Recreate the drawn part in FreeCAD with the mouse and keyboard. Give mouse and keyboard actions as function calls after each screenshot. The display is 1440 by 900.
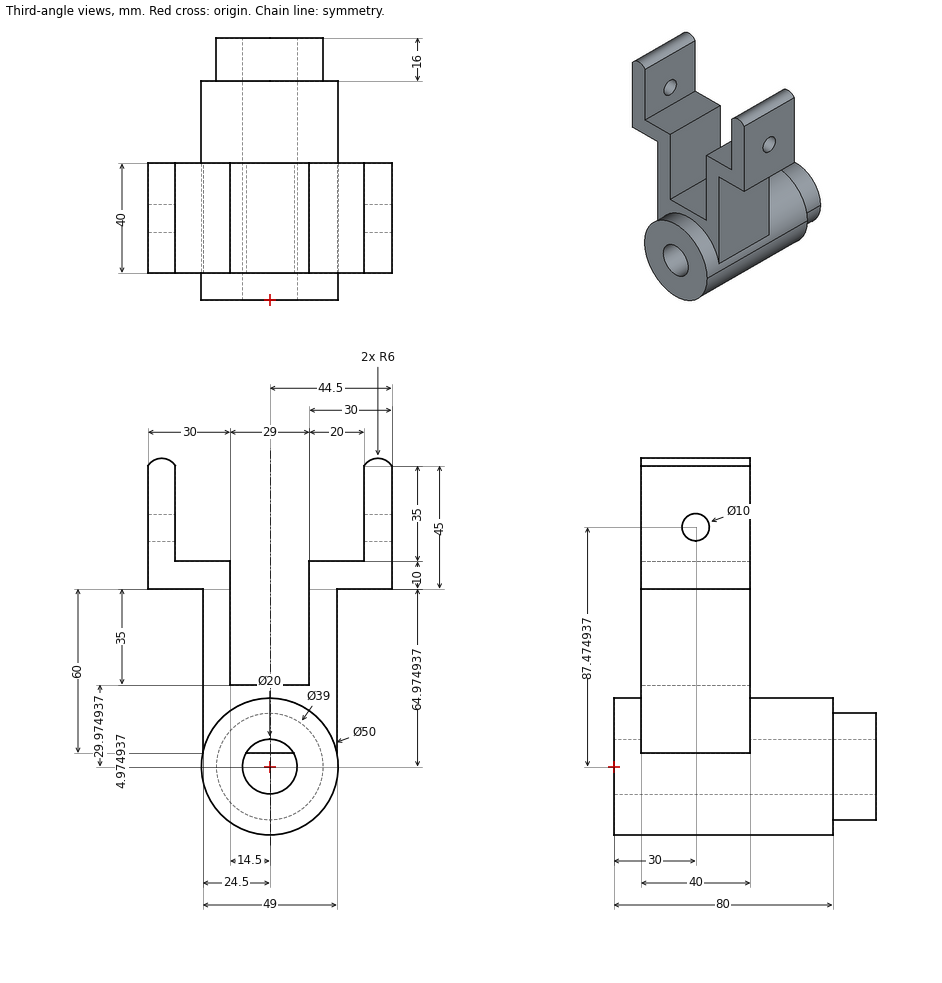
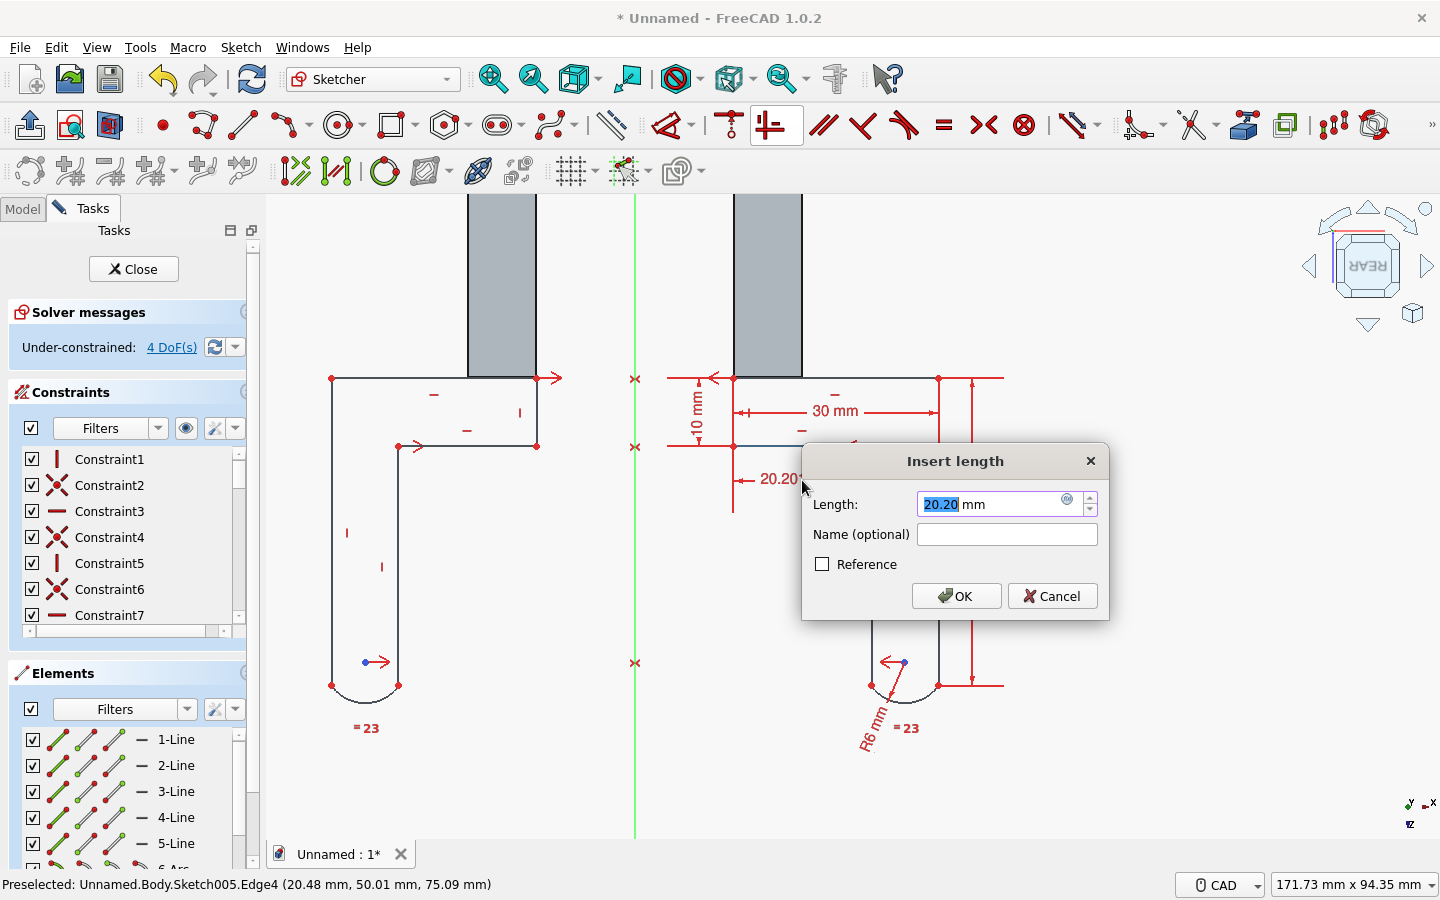
text(20)
key(Return)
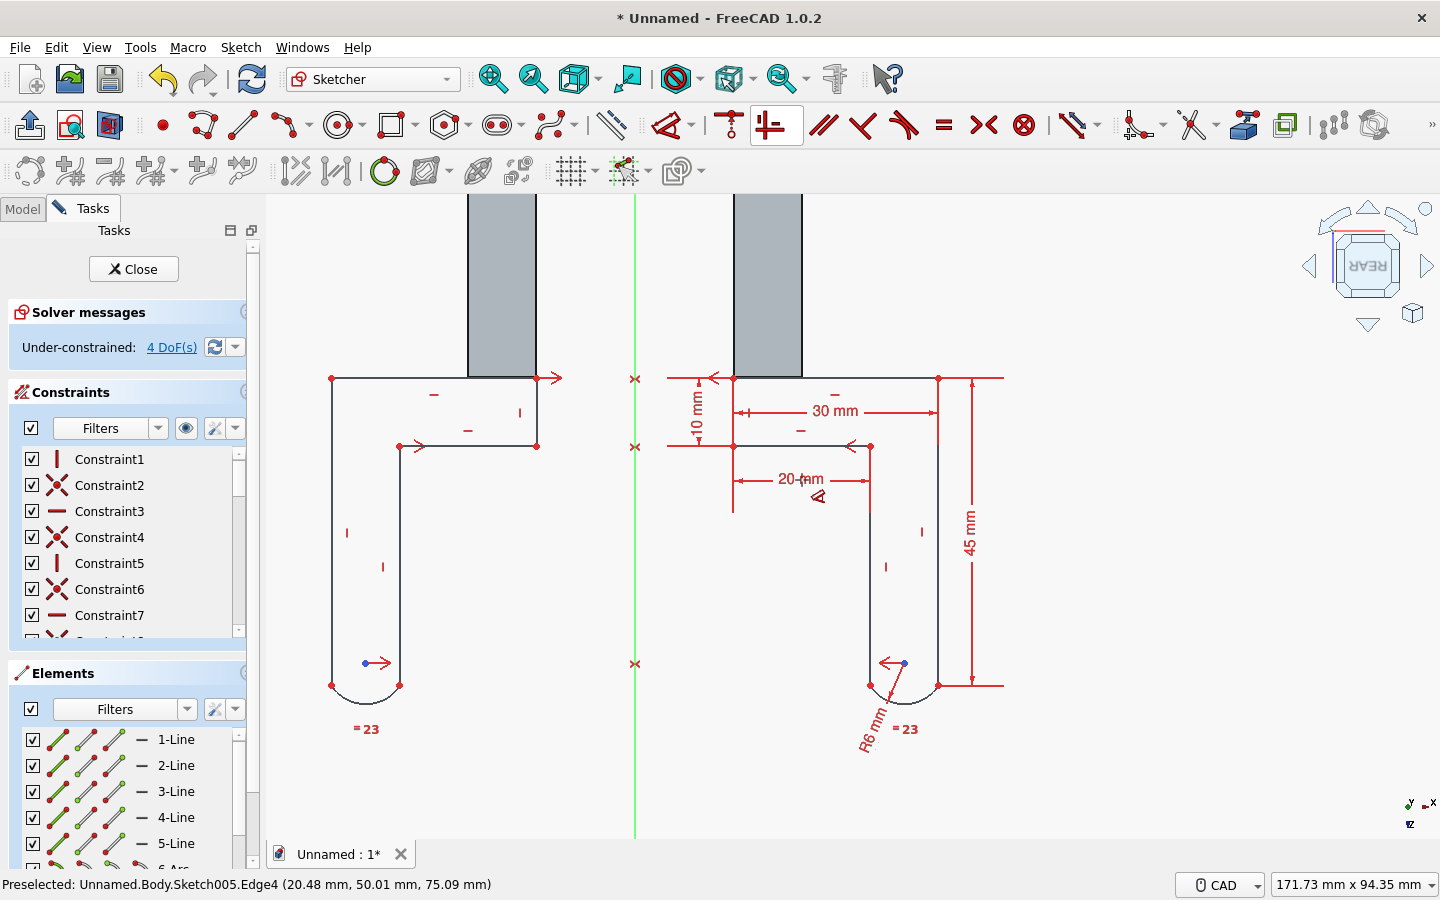
click(870, 518)
click(904, 566)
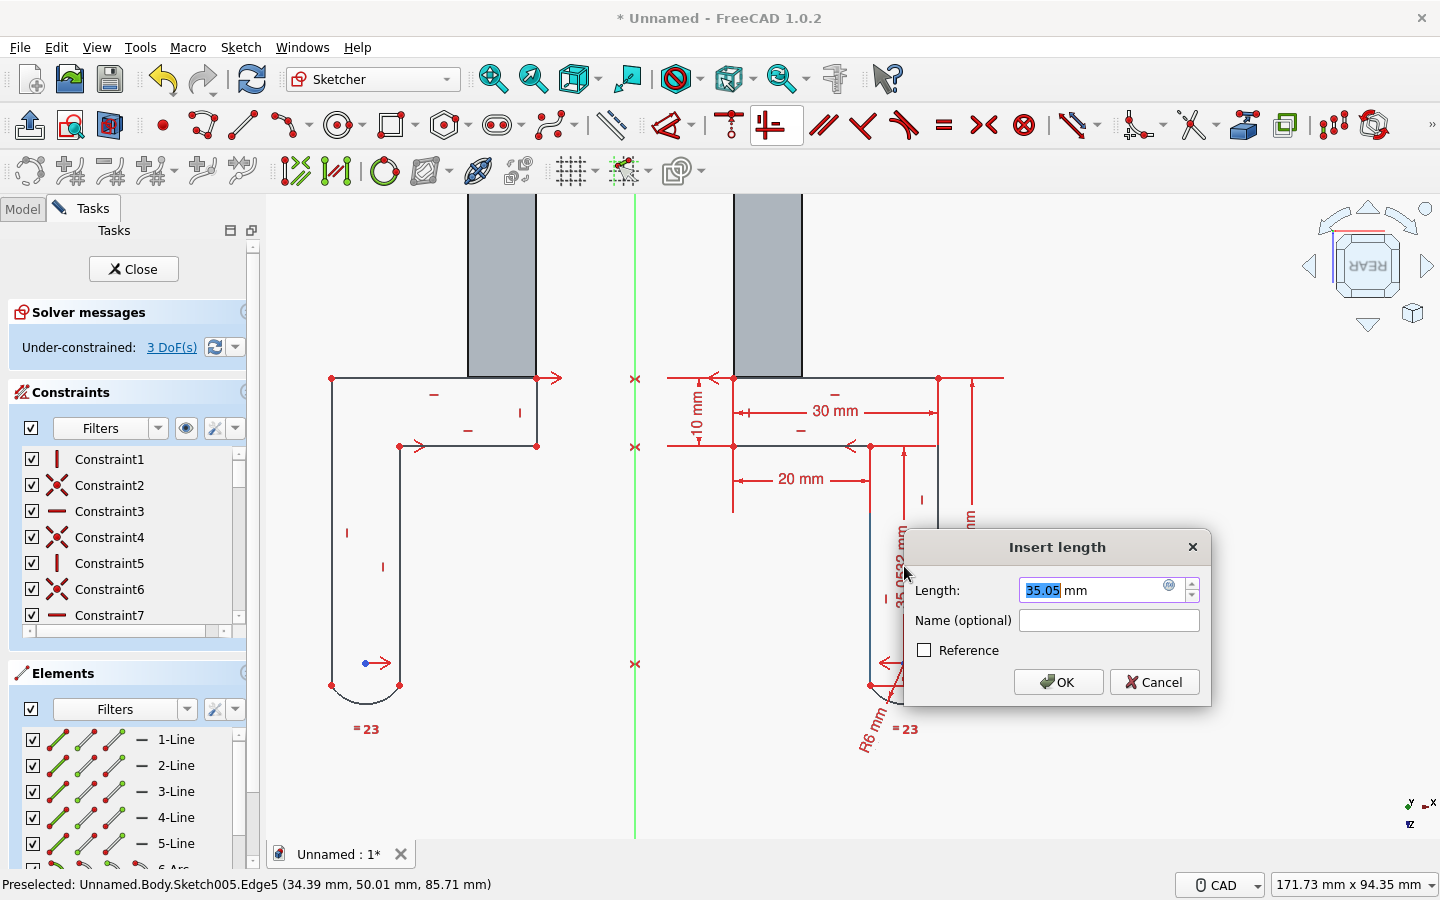
text(35)
key(Return)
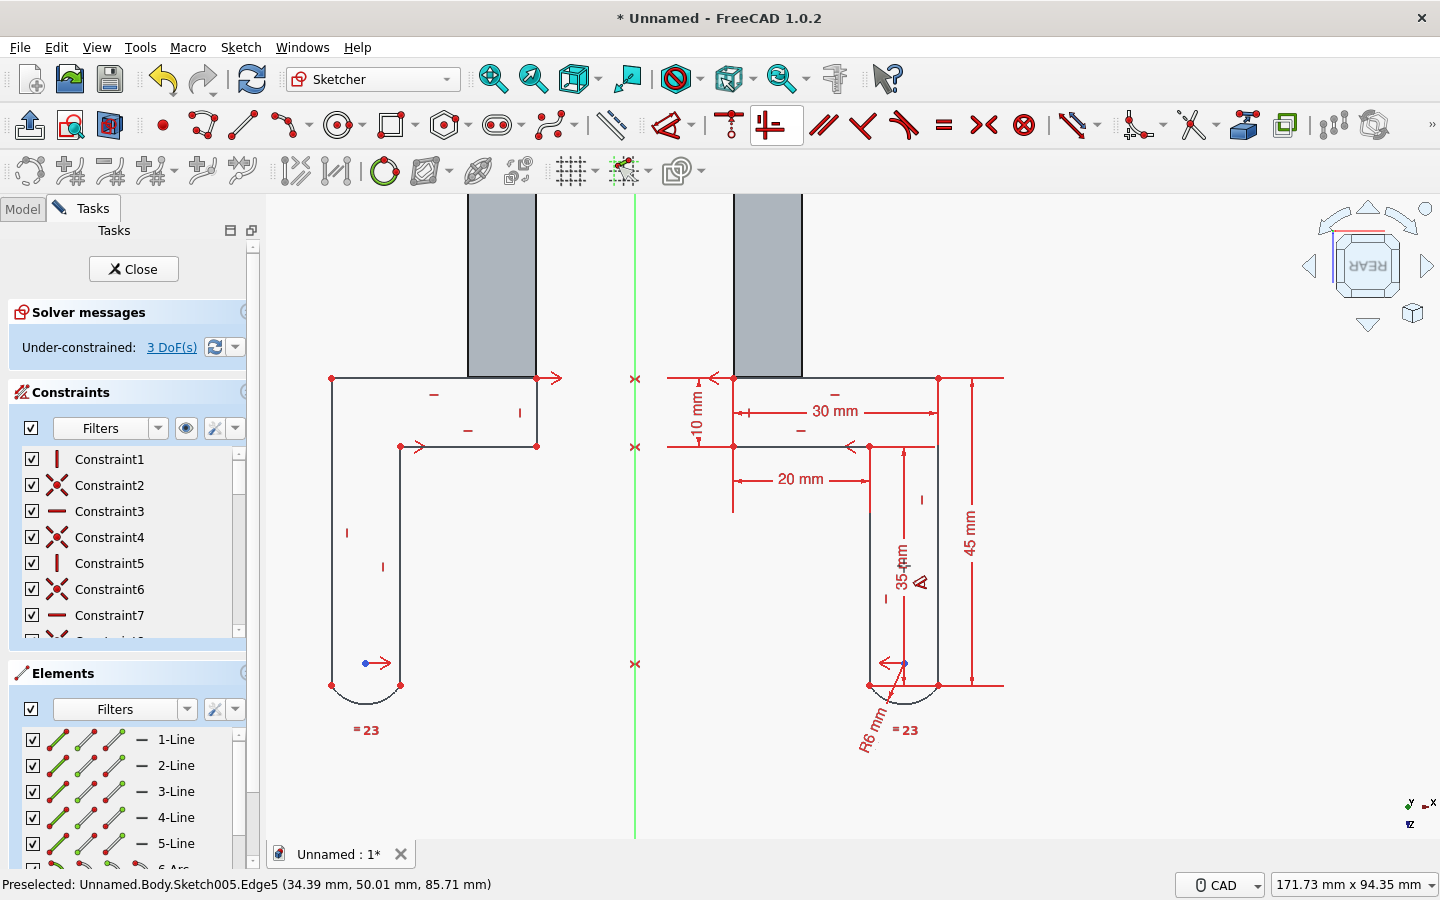
click(475, 378)
click(434, 412)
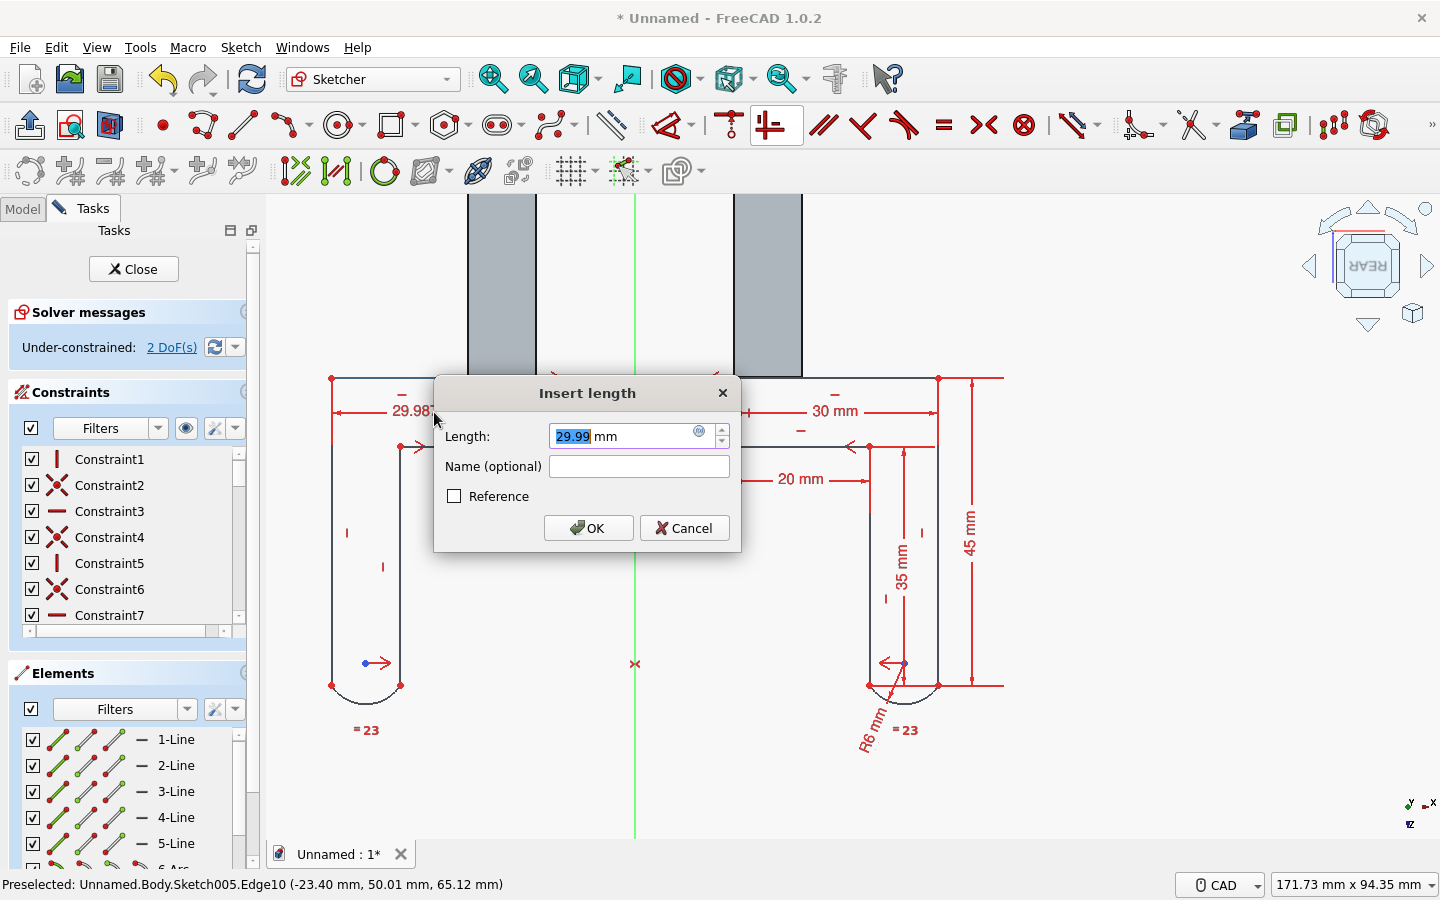
text(30)
key(Return)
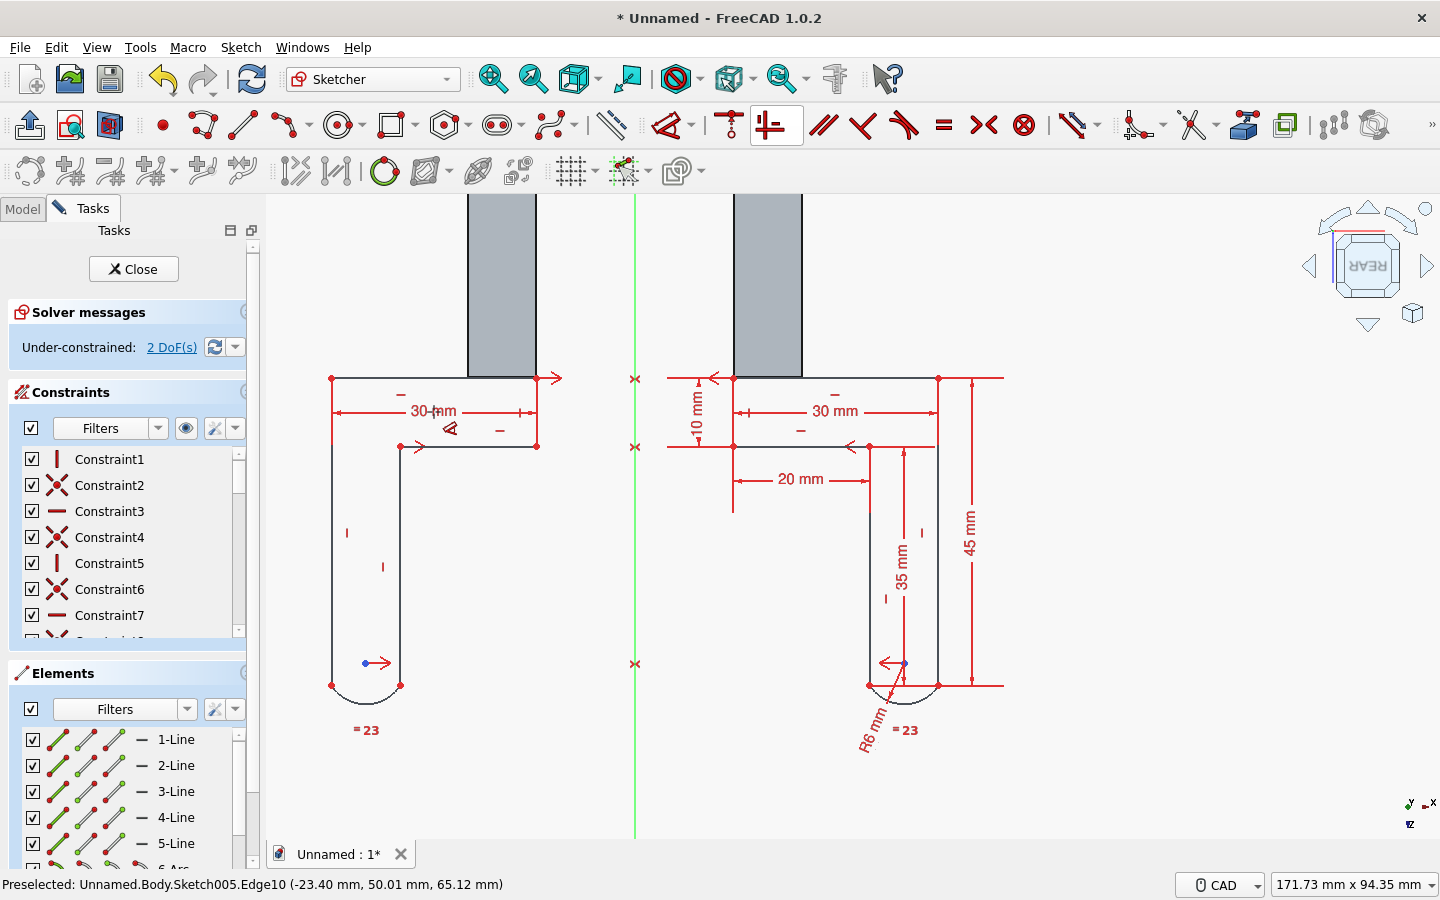
click(938, 686)
click(787, 720)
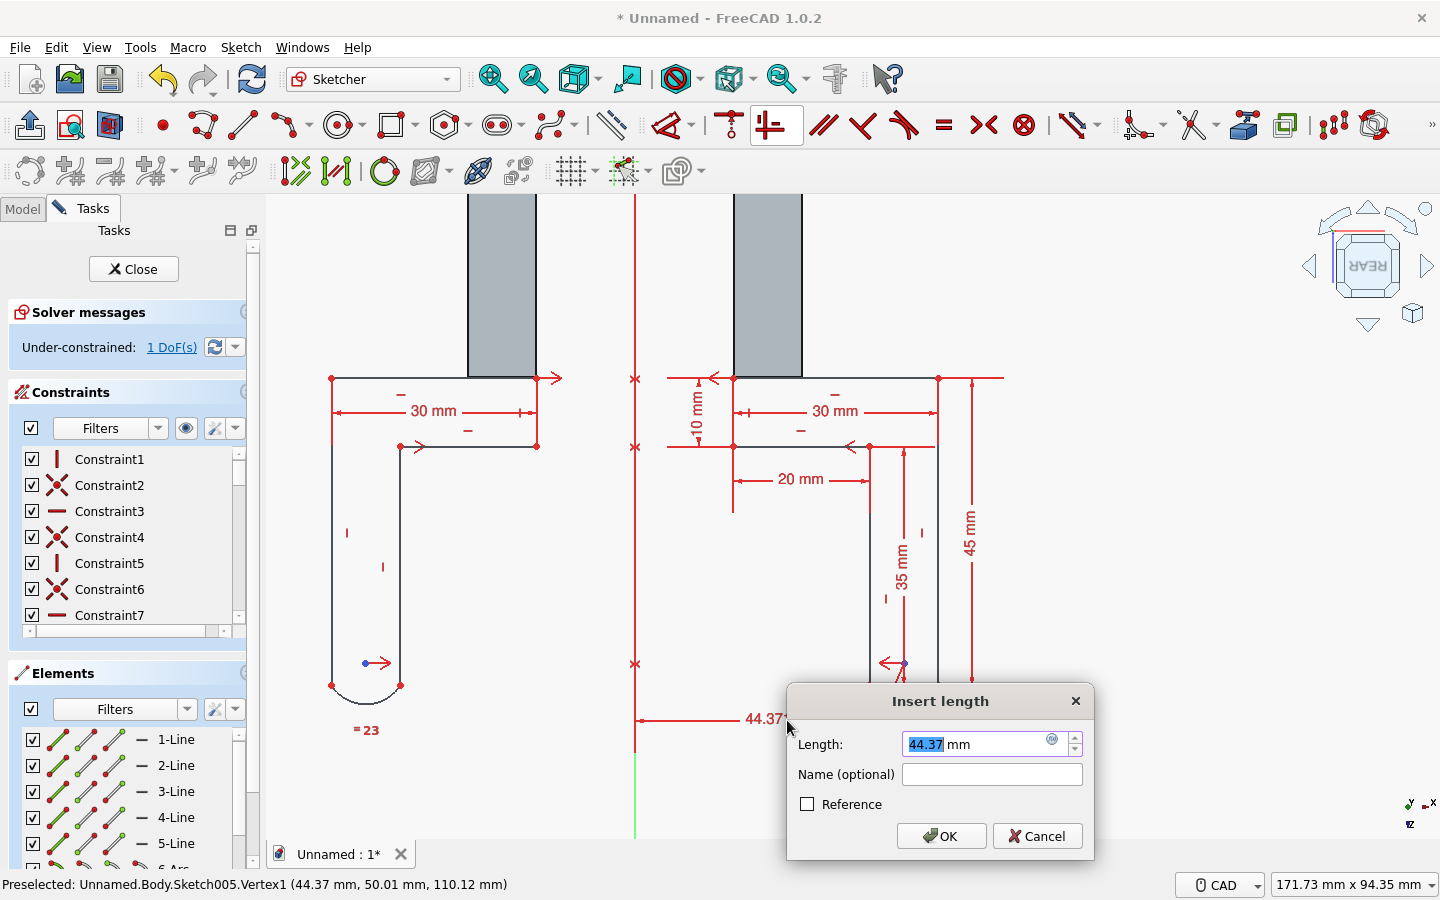
text(44.5)
key(Return)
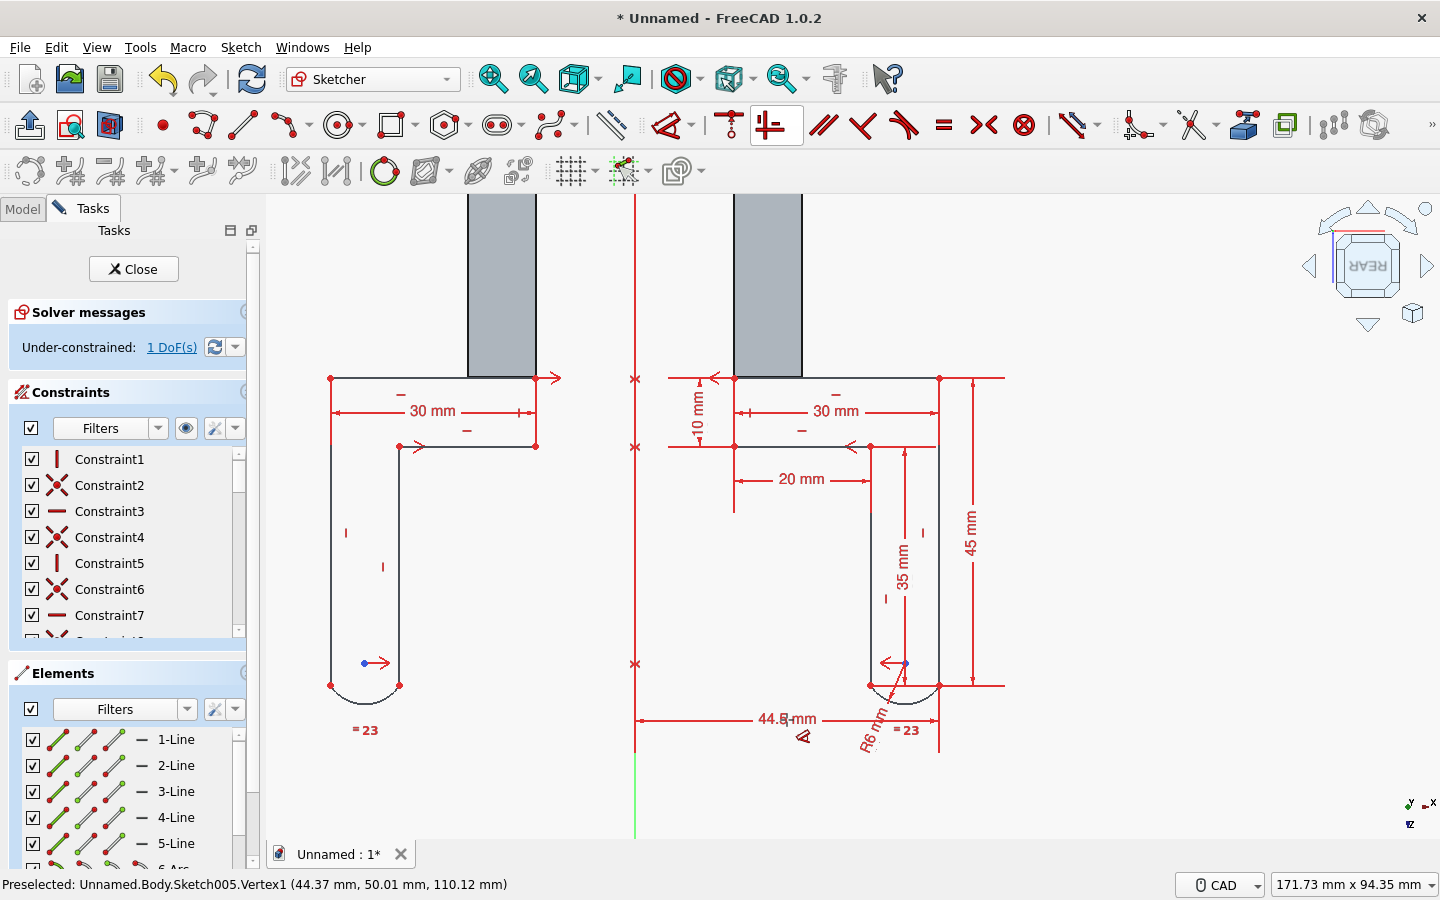
click(939, 378)
click(973, 300)